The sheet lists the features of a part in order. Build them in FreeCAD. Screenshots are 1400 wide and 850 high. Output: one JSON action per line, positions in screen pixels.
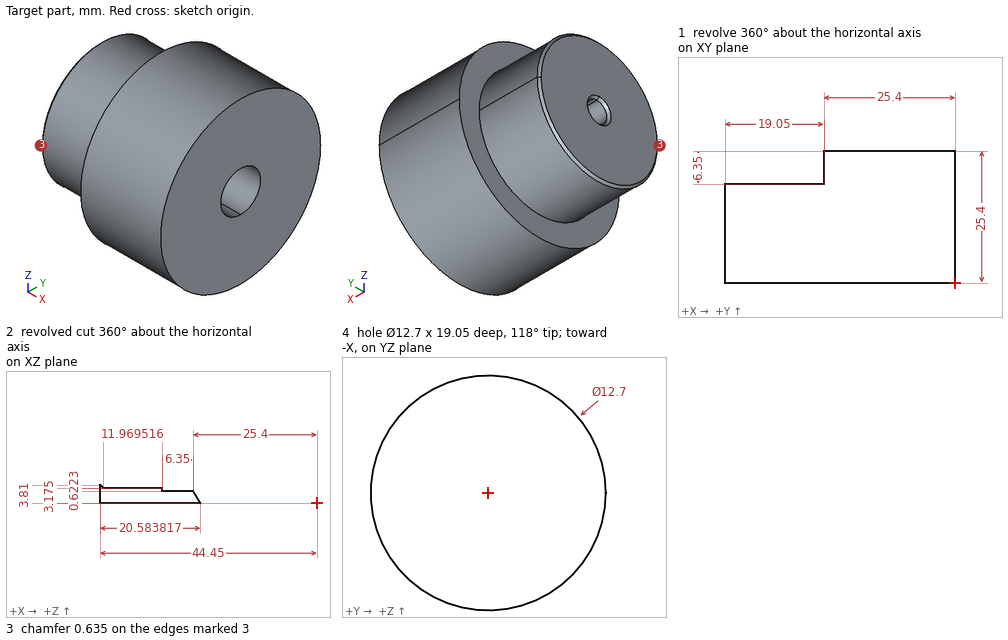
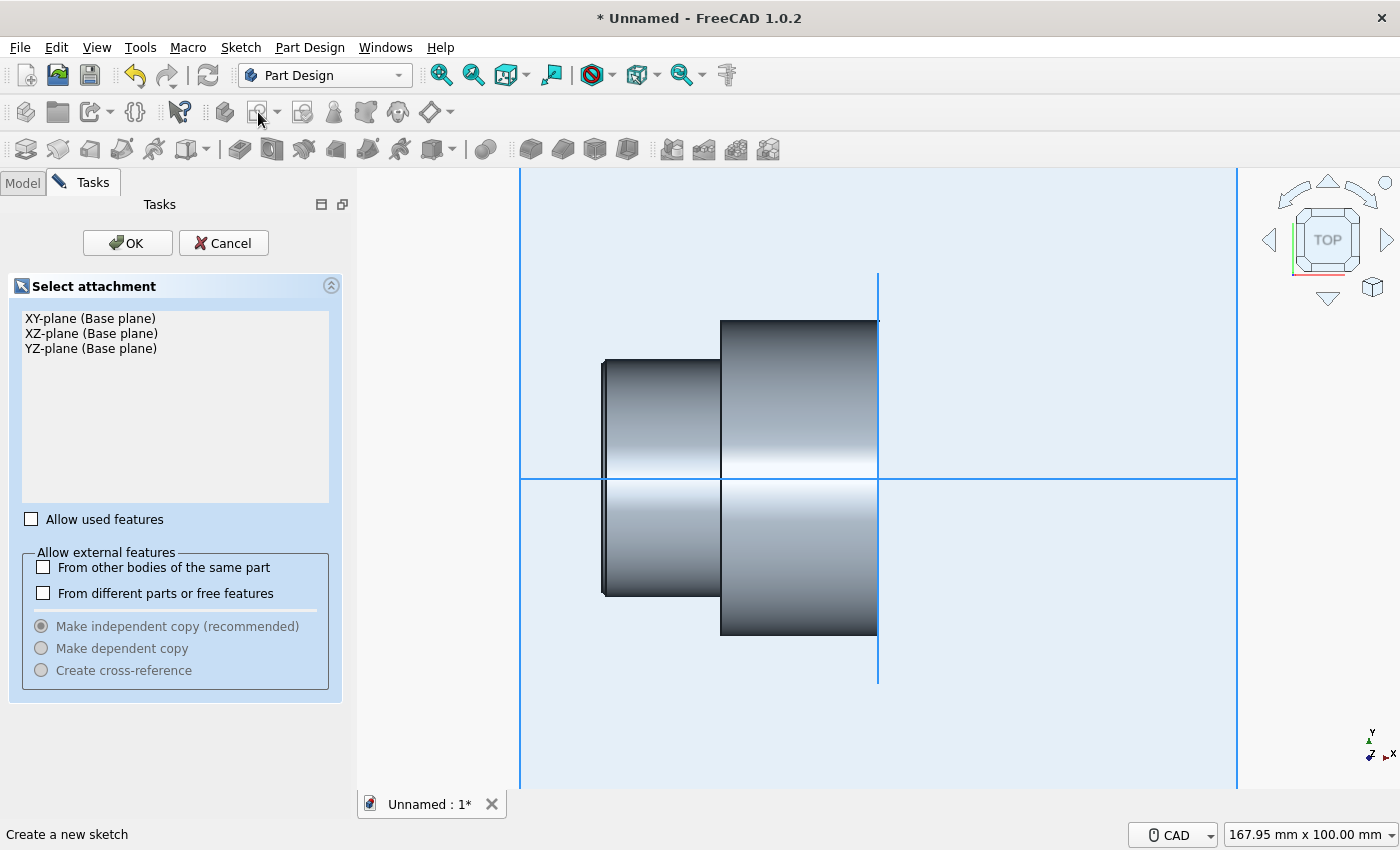
{"action": "left_click", "coordinate": [82, 348]}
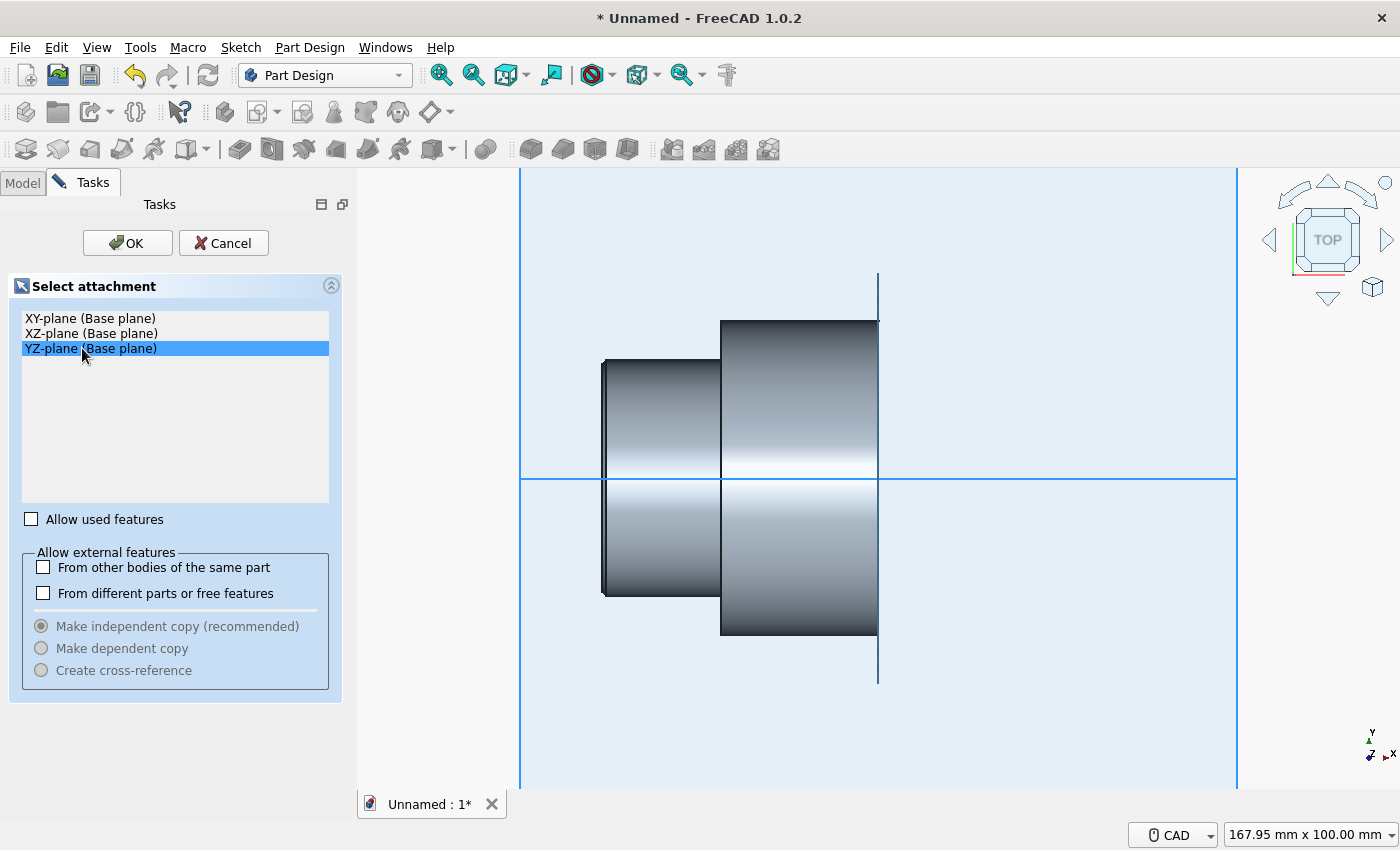
{"action": "left_click", "coordinate": [128, 243]}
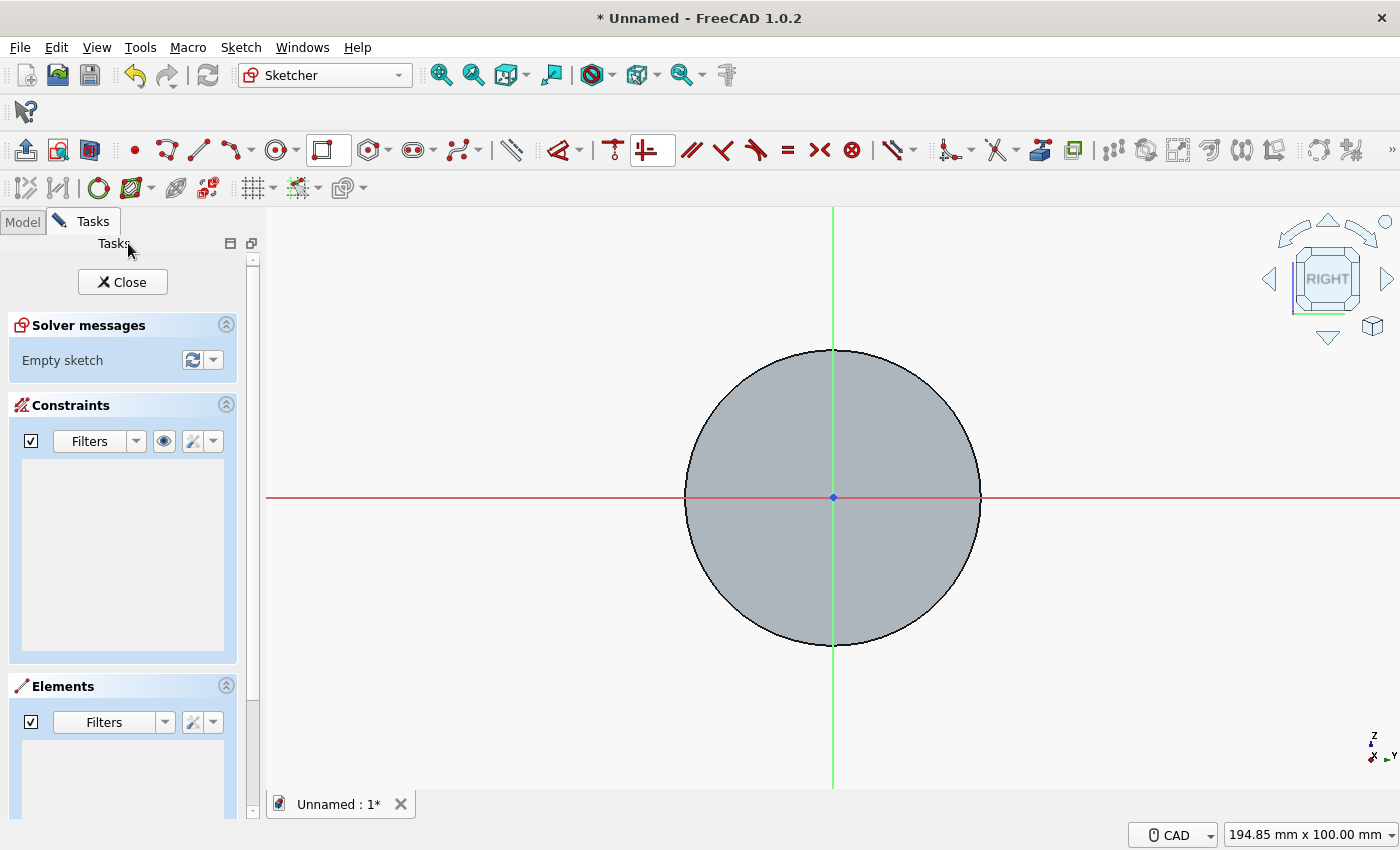
{"action": "scroll", "coordinate": [850, 498], "scroll_direction": "up", "scroll_amount": 8}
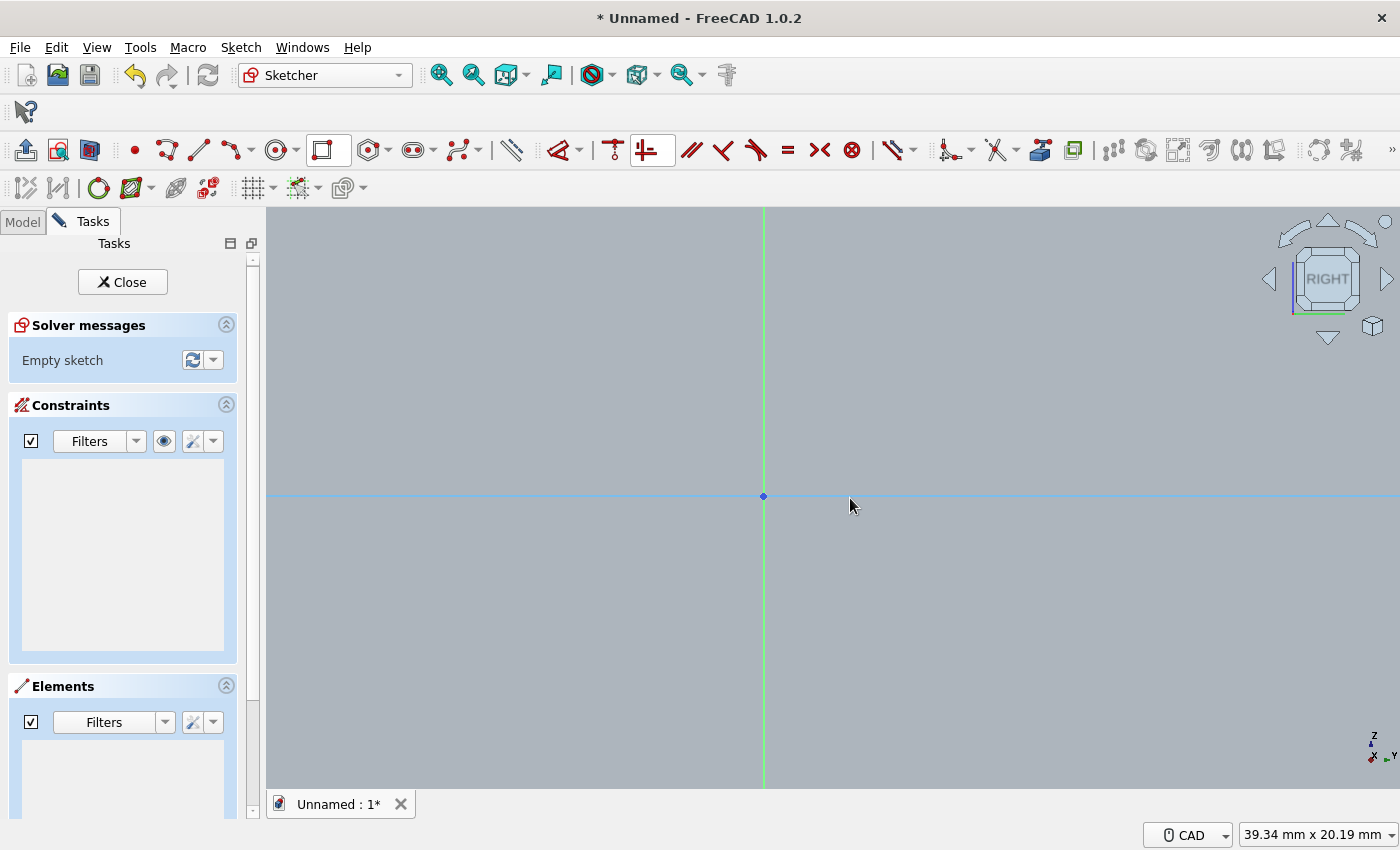
{"action": "left_click", "coordinate": [276, 150]}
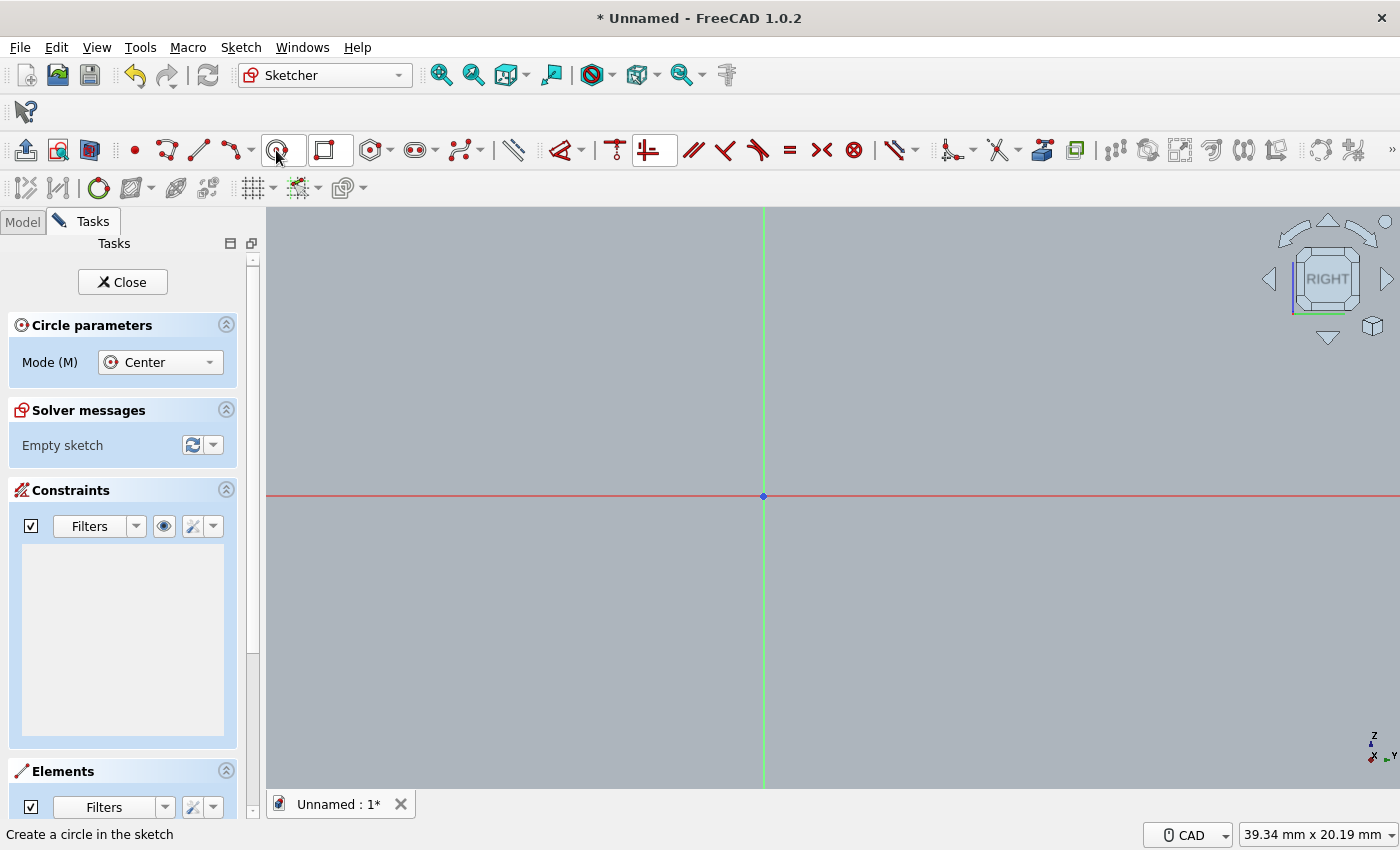
{"action": "left_click", "coordinate": [764, 496]}
{"action": "left_click", "coordinate": [893, 367]}
{"action": "key", "text": "Escape"}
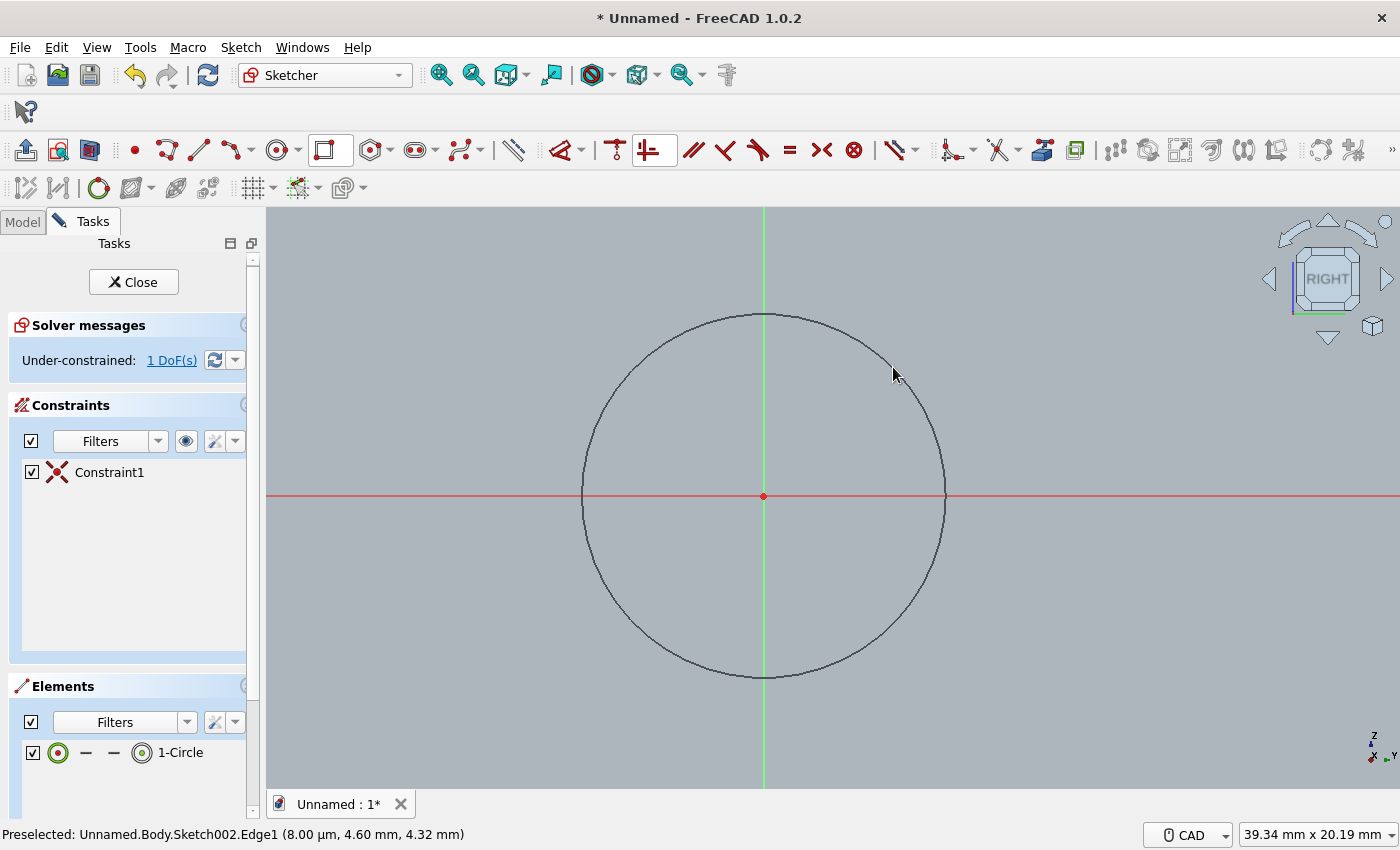
{"action": "left_click", "coordinate": [560, 150]}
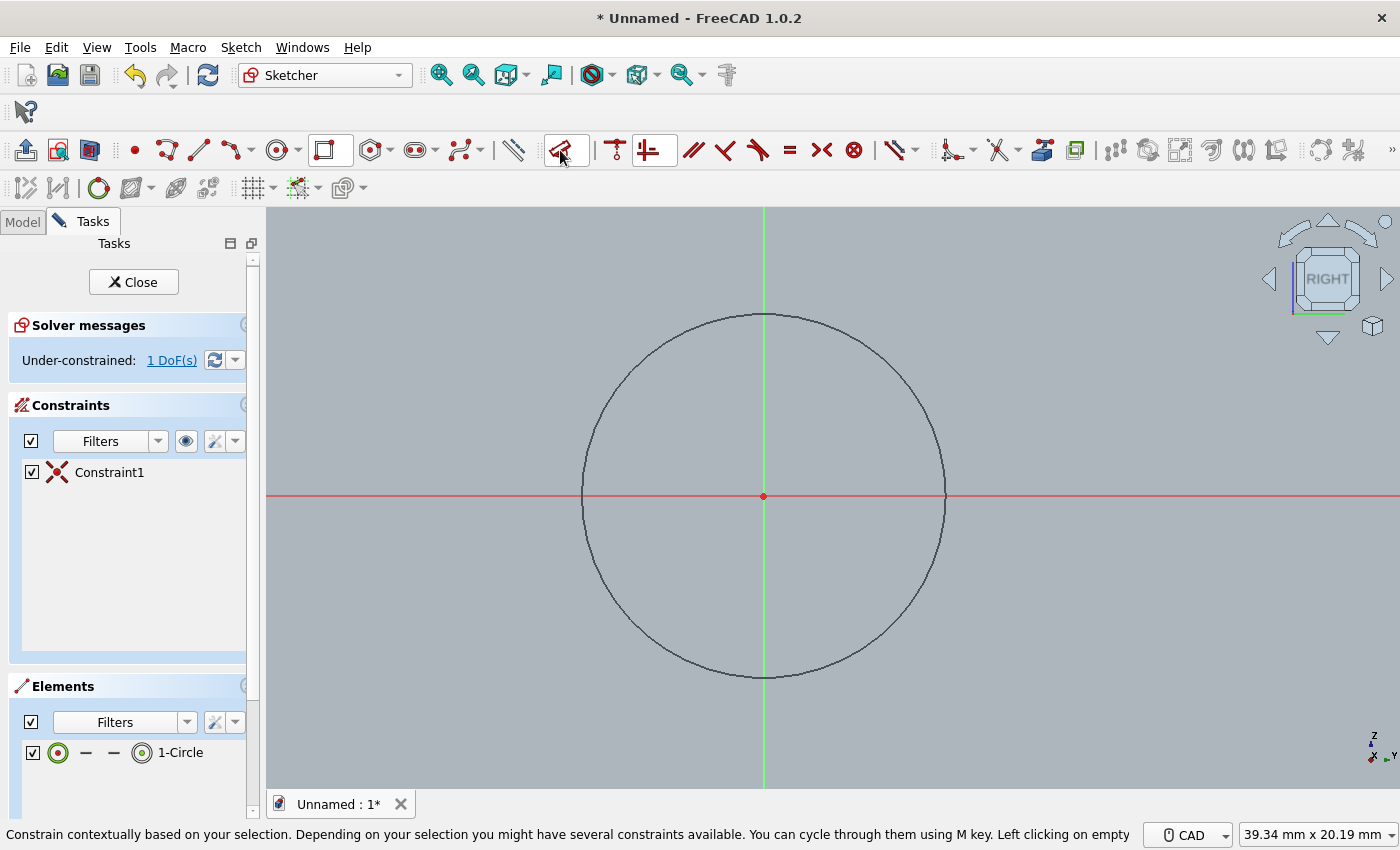
{"action": "left_click", "coordinate": [892, 367]}
{"action": "left_click", "coordinate": [915, 344]}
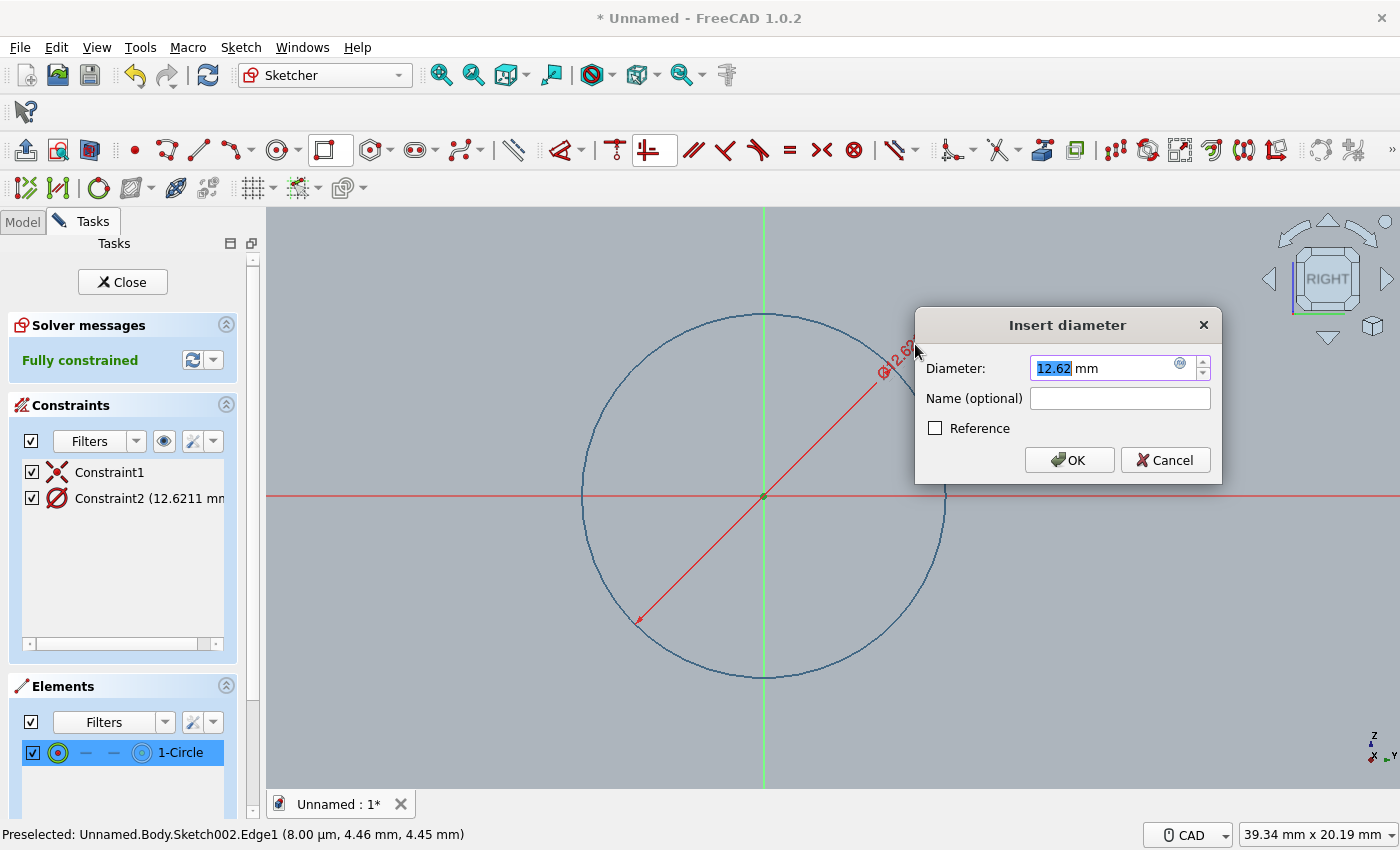
{"action": "type", "text": "12.7"}
{"action": "key", "text": "Return"}
{"action": "key", "text": "Escape"}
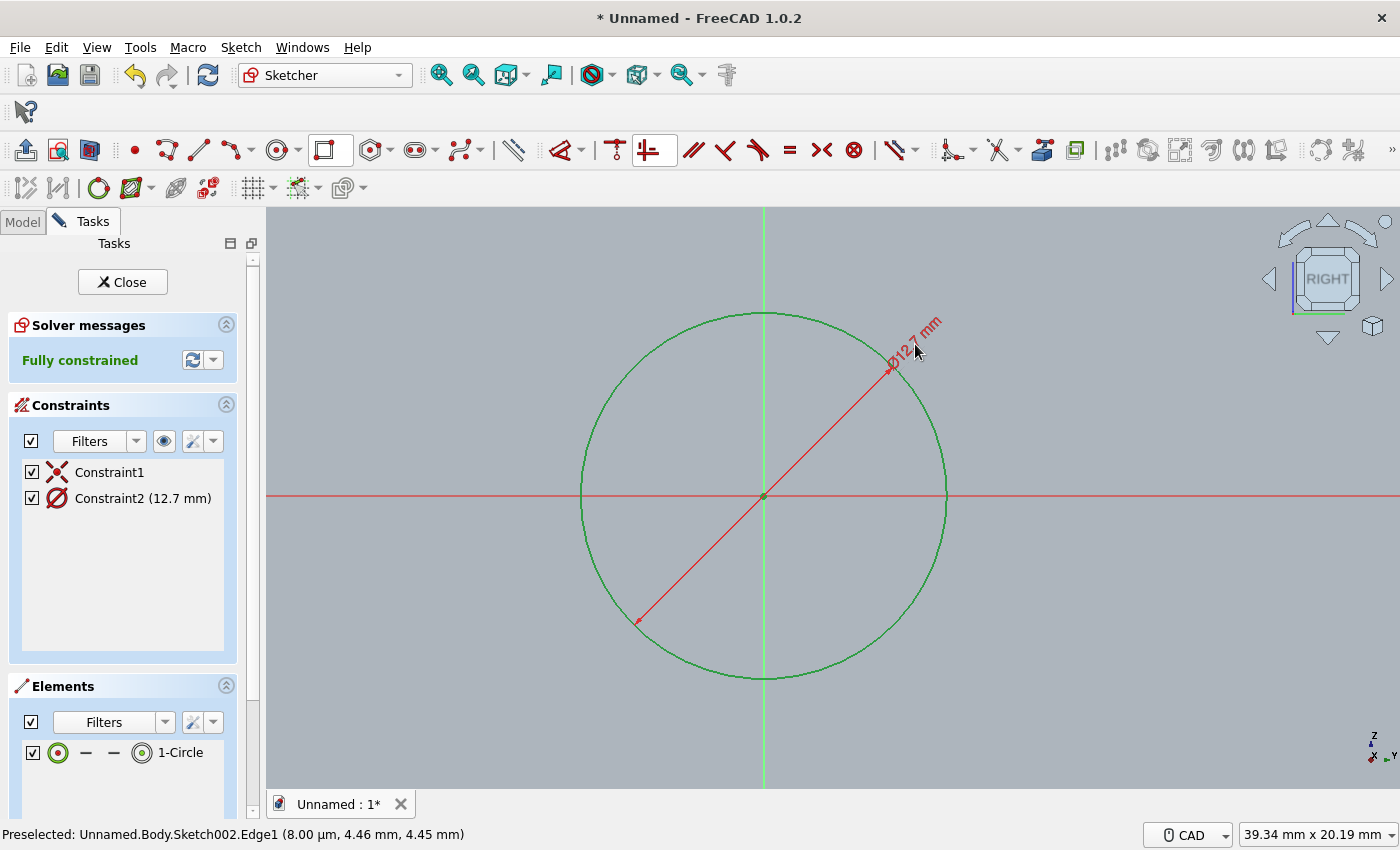
{"action": "left_click", "coordinate": [123, 282]}